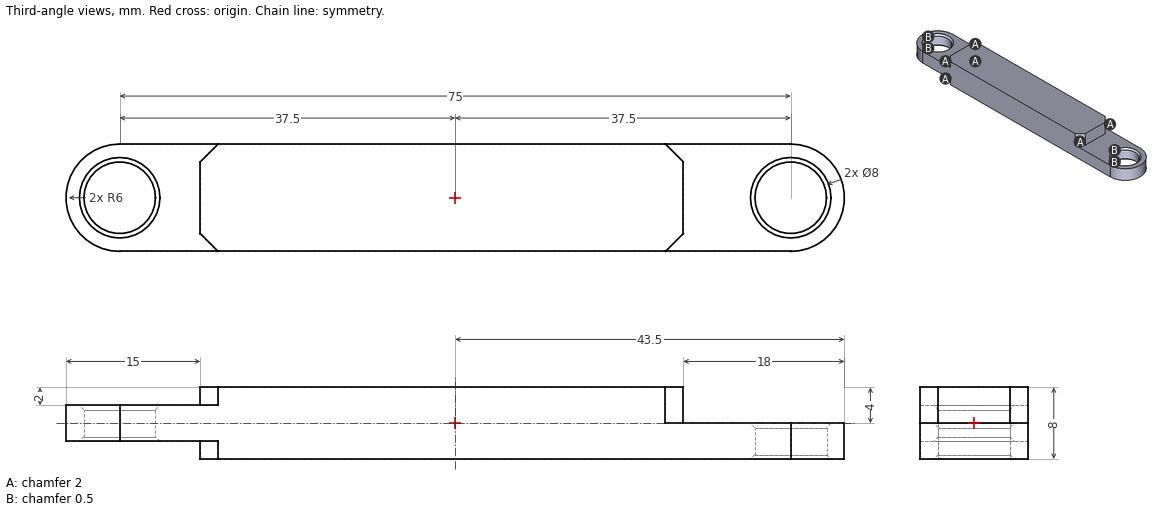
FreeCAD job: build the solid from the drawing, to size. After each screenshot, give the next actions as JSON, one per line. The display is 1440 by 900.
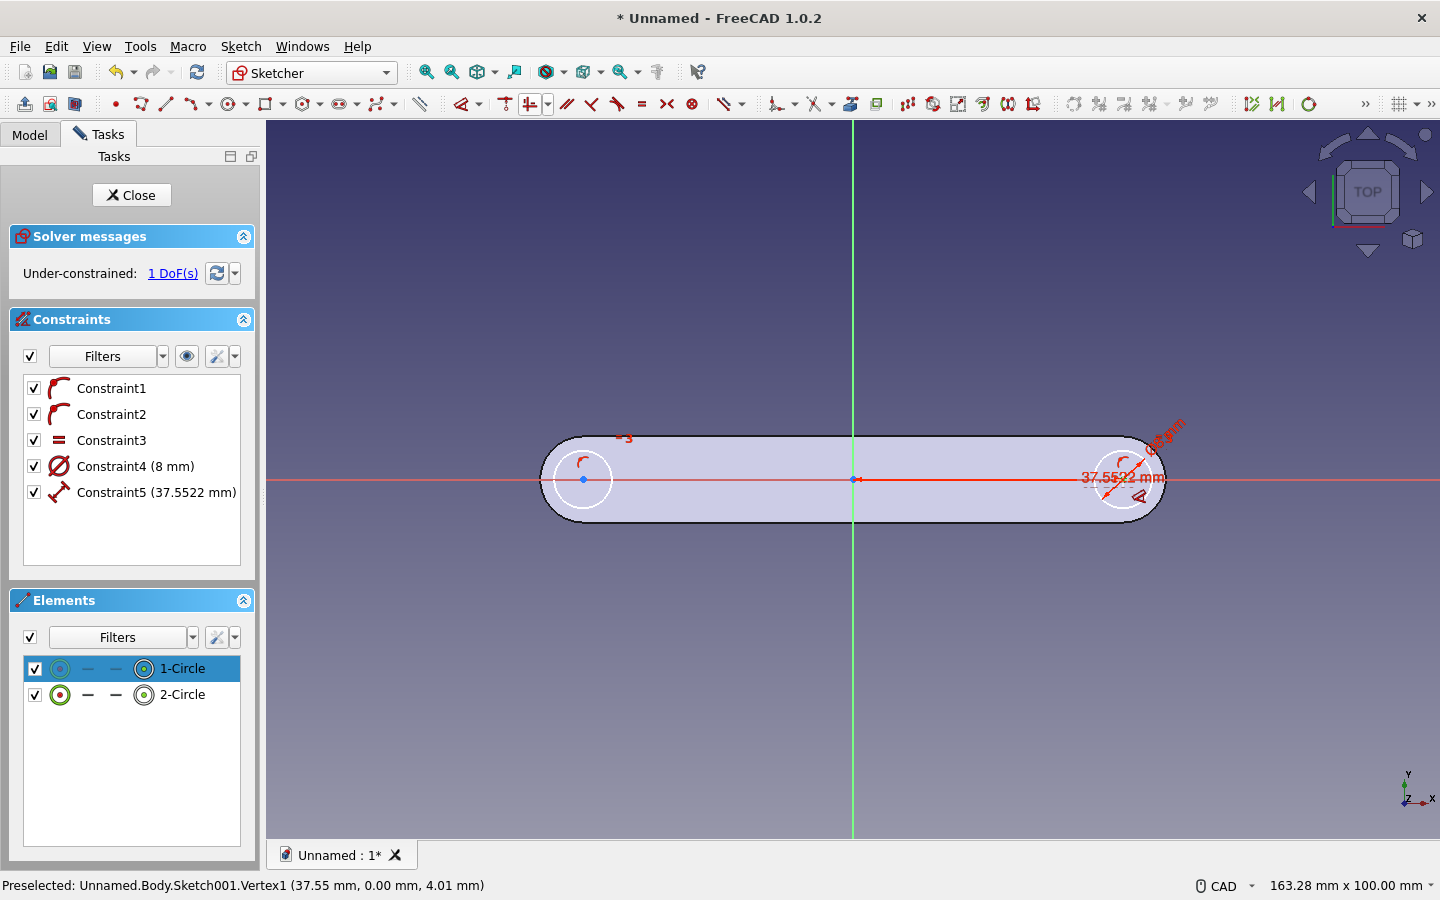
{"action": "left_click", "coordinate": [583, 480]}
{"action": "left_click", "coordinate": [729, 514]}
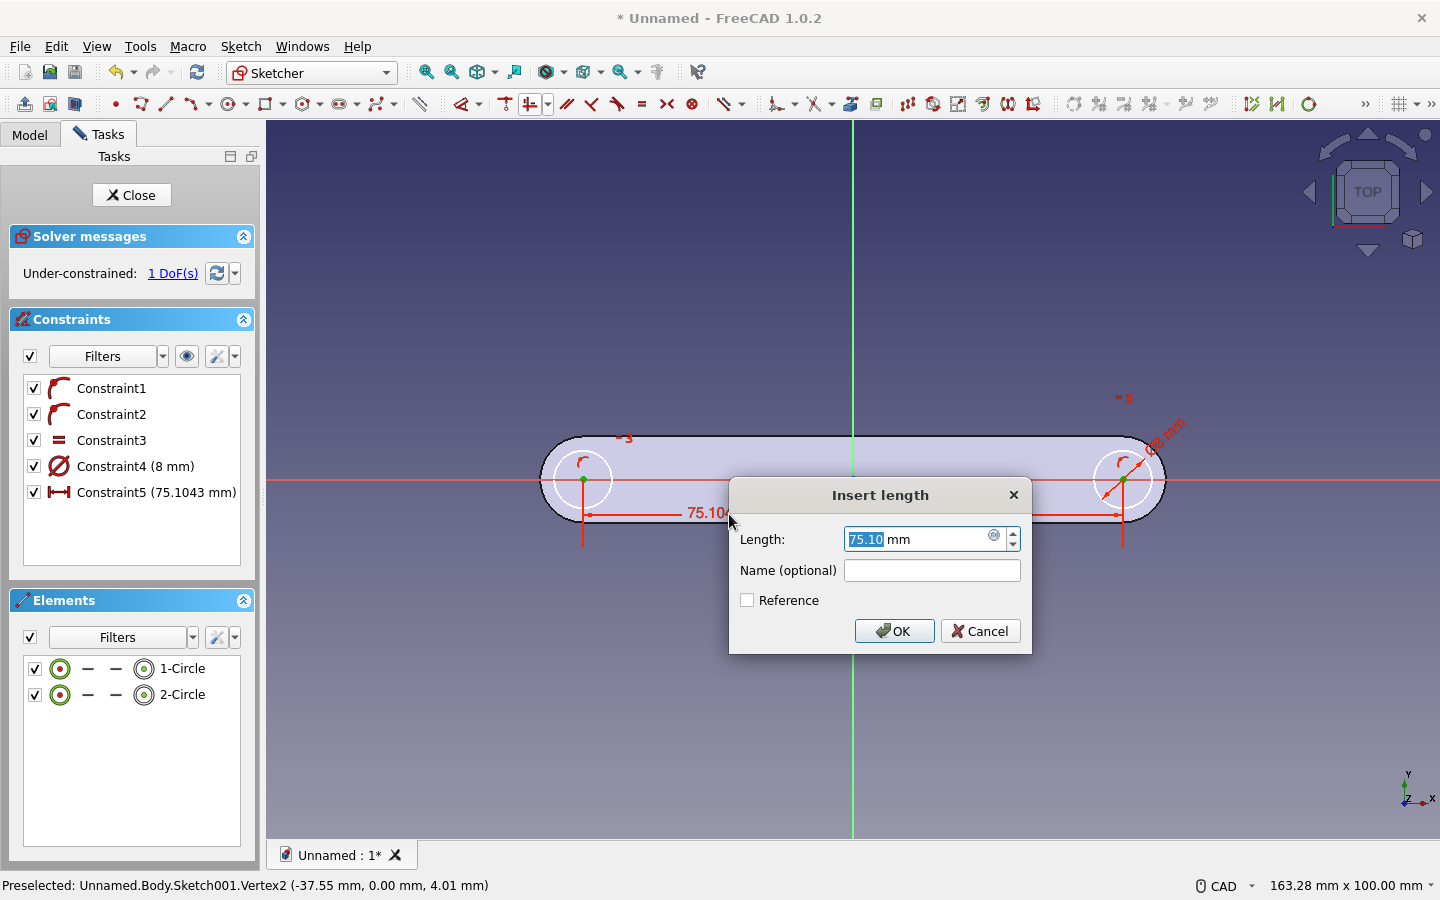
{"action": "type", "text": "75"}
{"action": "key", "text": "Return"}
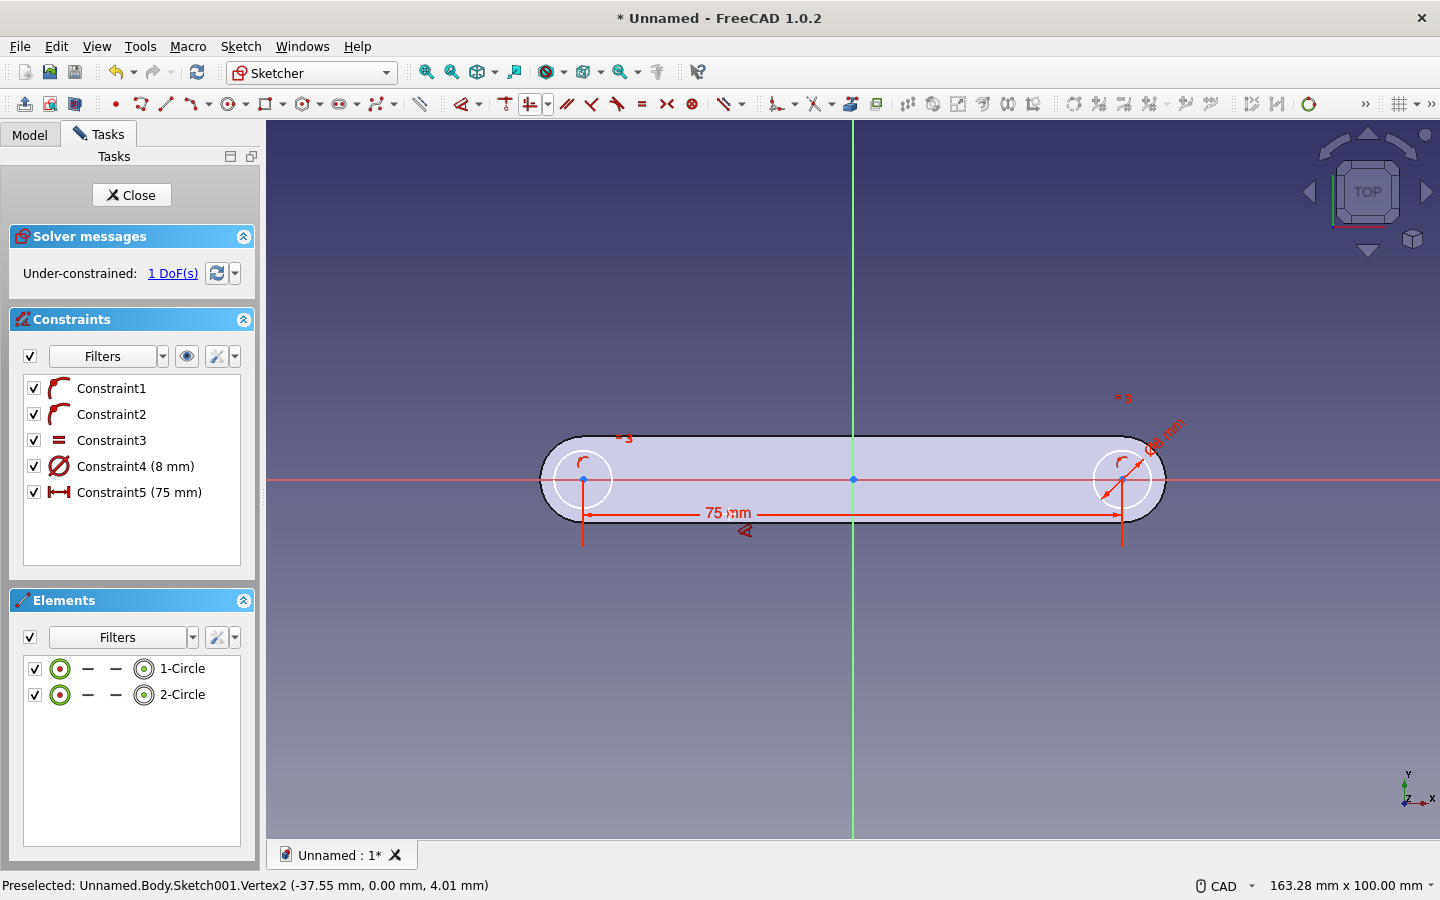
{"action": "left_click", "coordinate": [1122, 480]}
{"action": "left_click", "coordinate": [988, 514]}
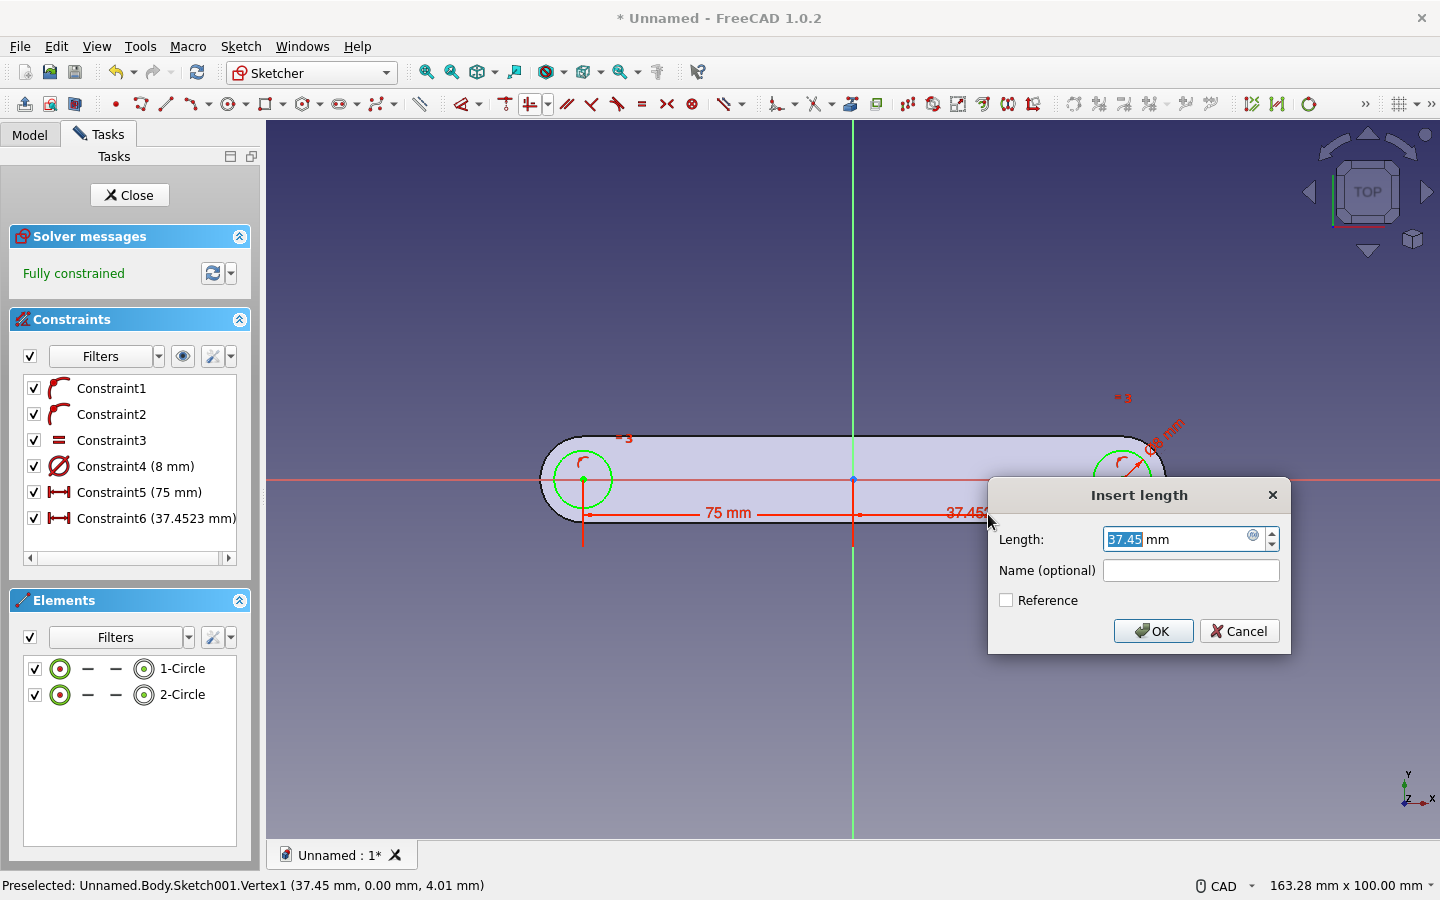
{"action": "type", "text": "37.5"}
{"action": "key", "text": "Return"}
{"action": "key", "text": "Escape"}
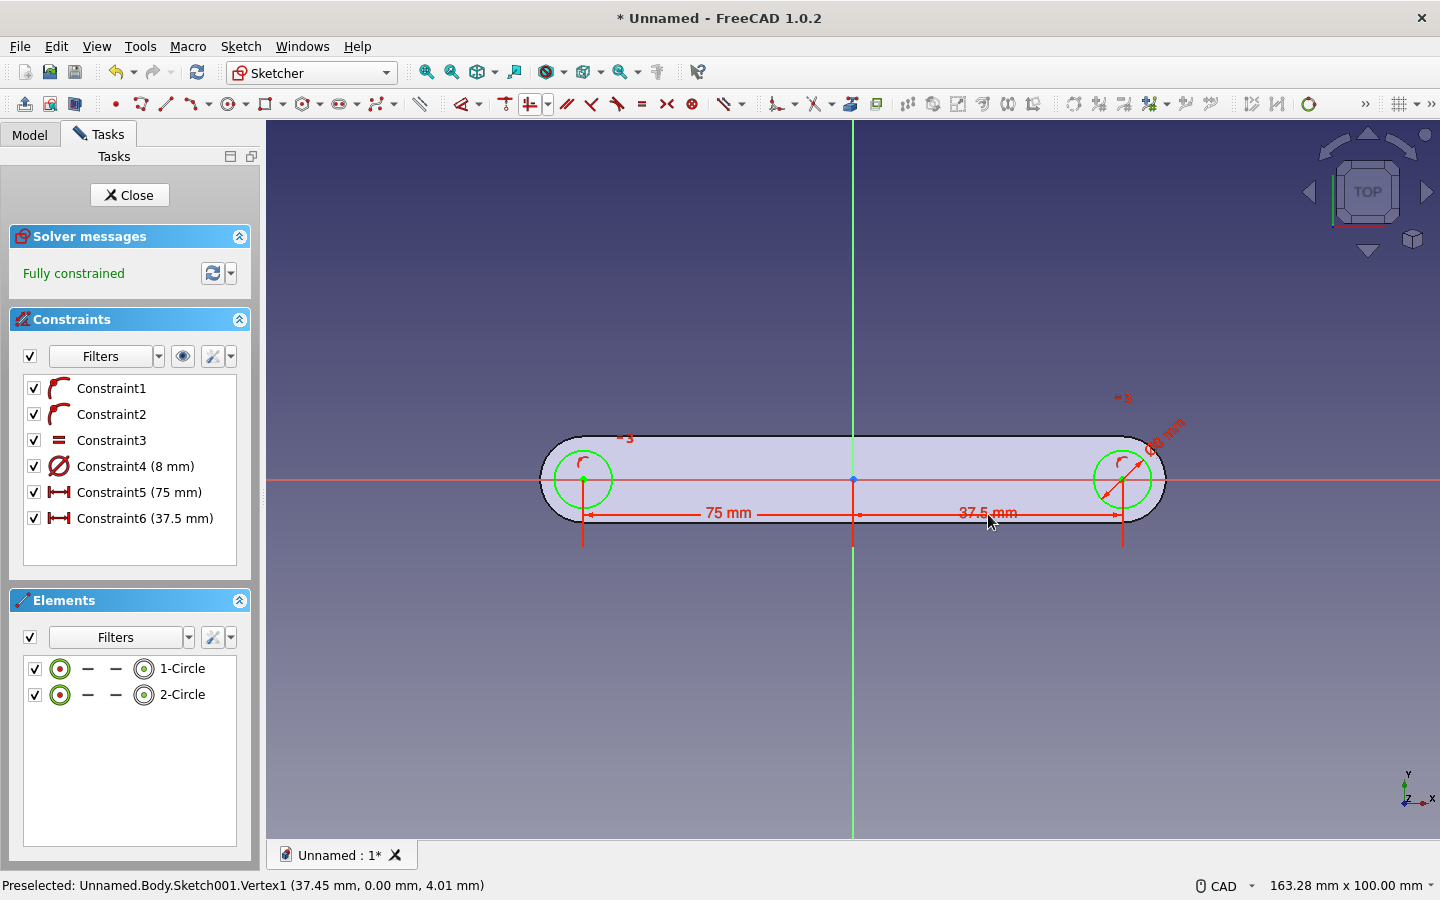
{"action": "left_click", "coordinate": [130, 195]}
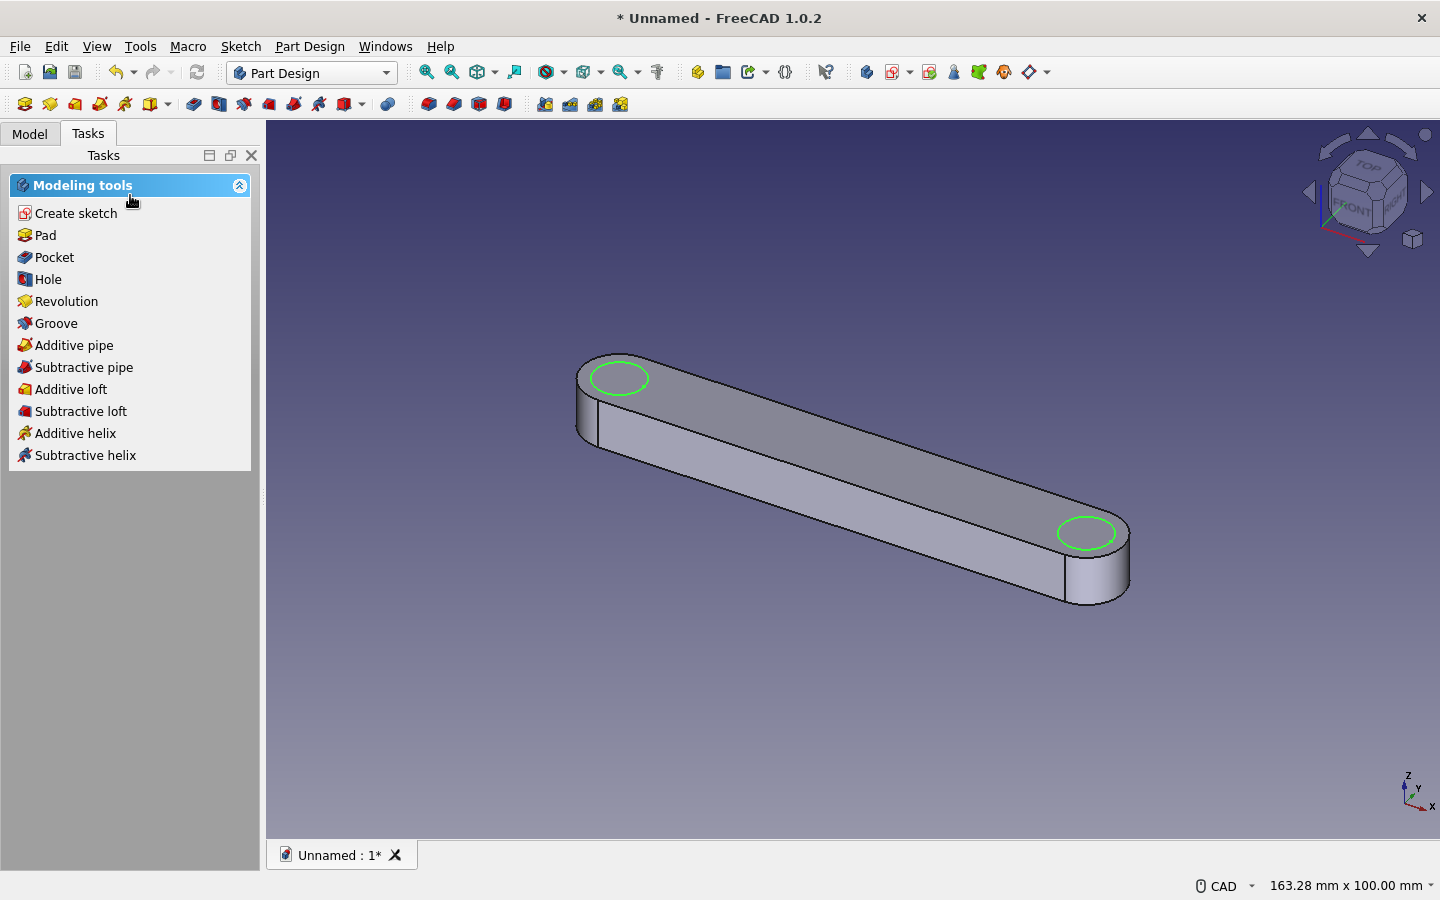
{"action": "left_click", "coordinate": [194, 104]}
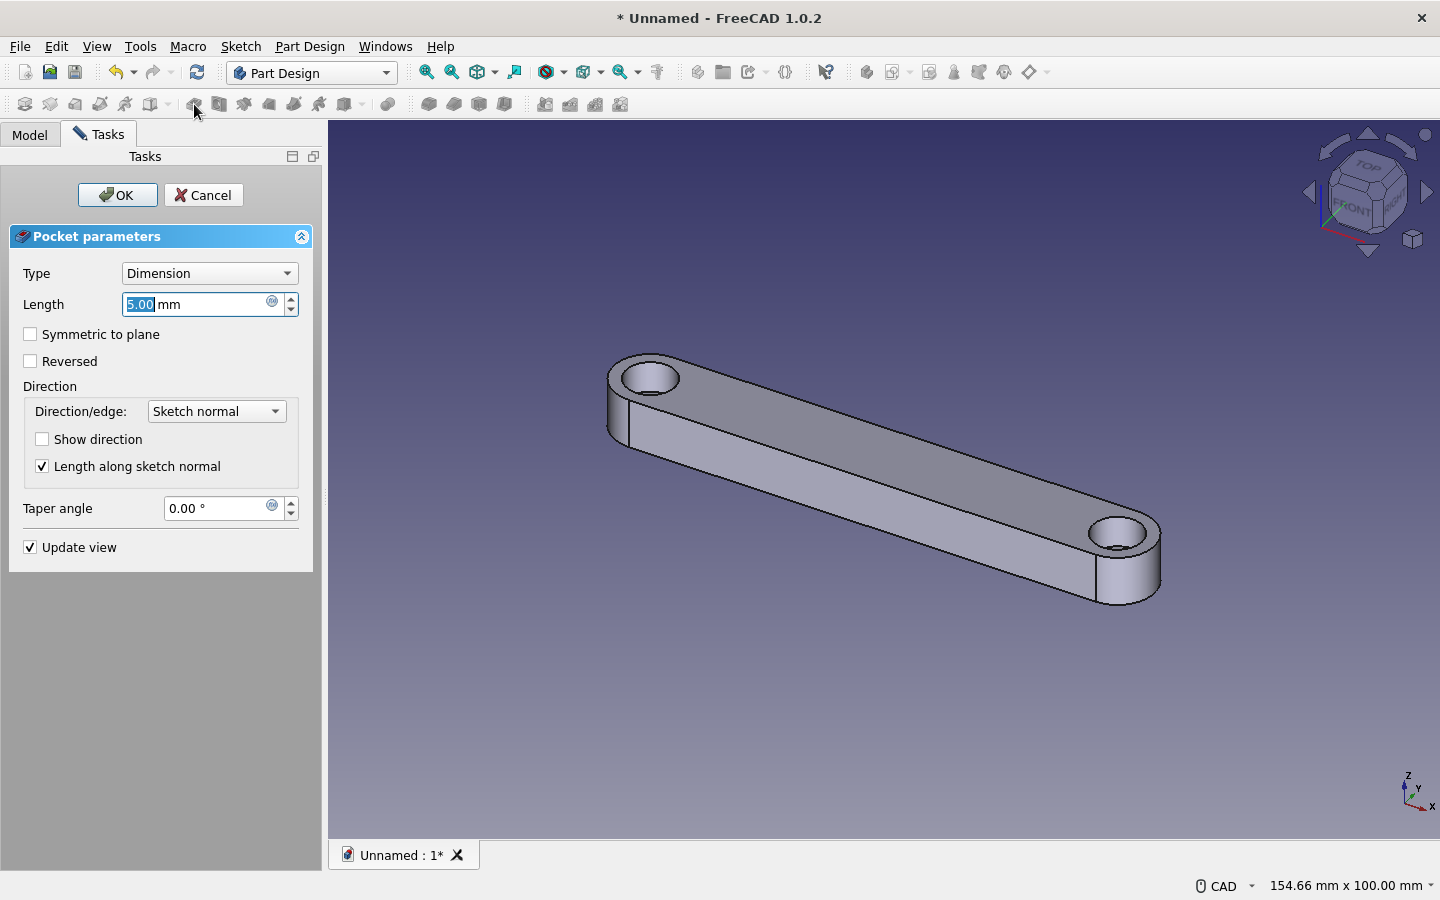
{"action": "left_click", "coordinate": [210, 274]}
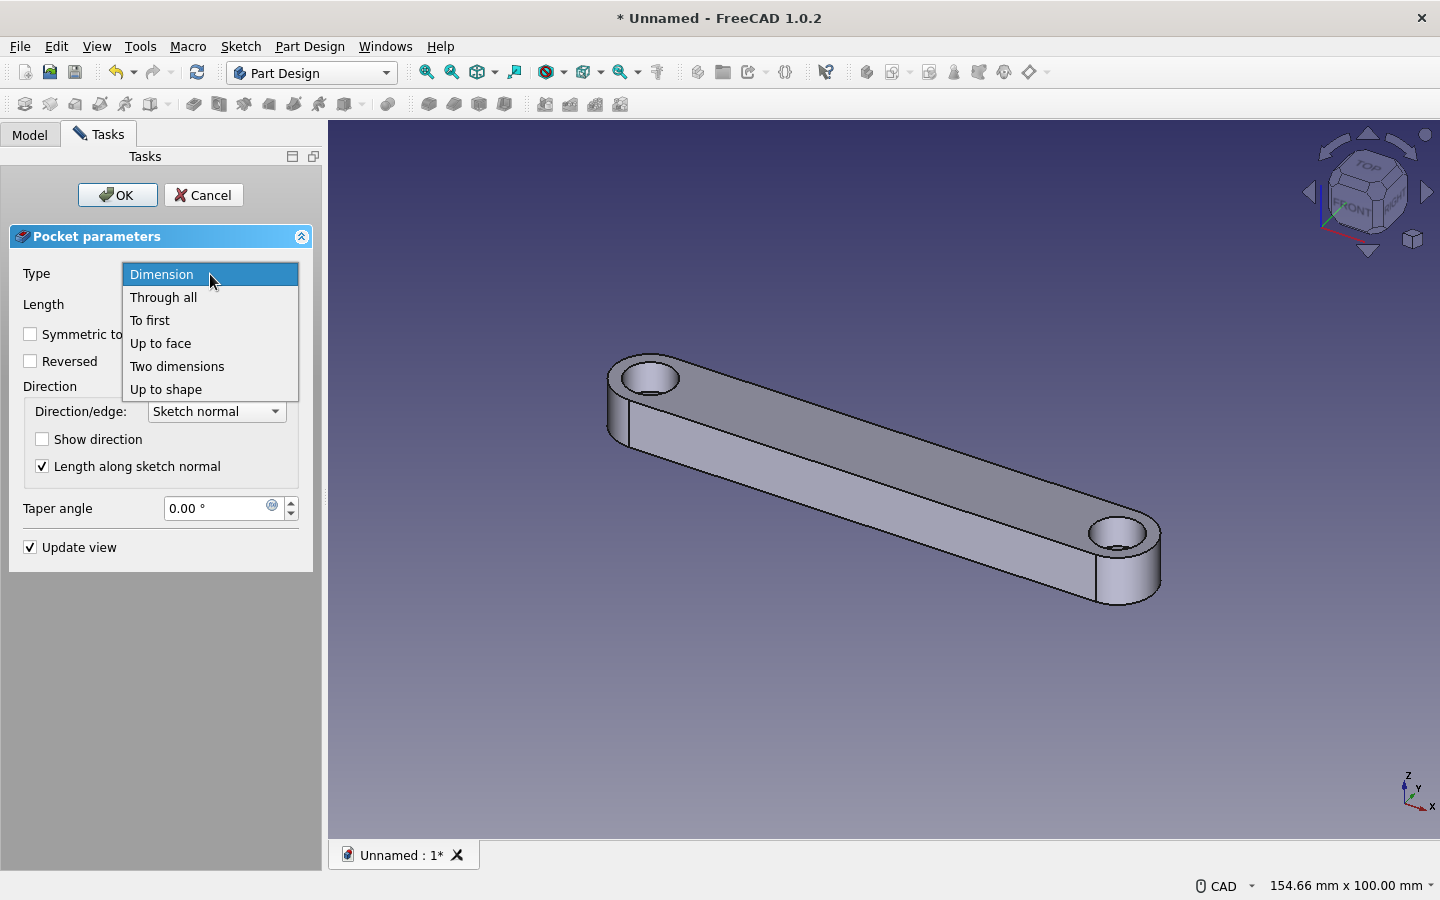
{"action": "left_click", "coordinate": [208, 298]}